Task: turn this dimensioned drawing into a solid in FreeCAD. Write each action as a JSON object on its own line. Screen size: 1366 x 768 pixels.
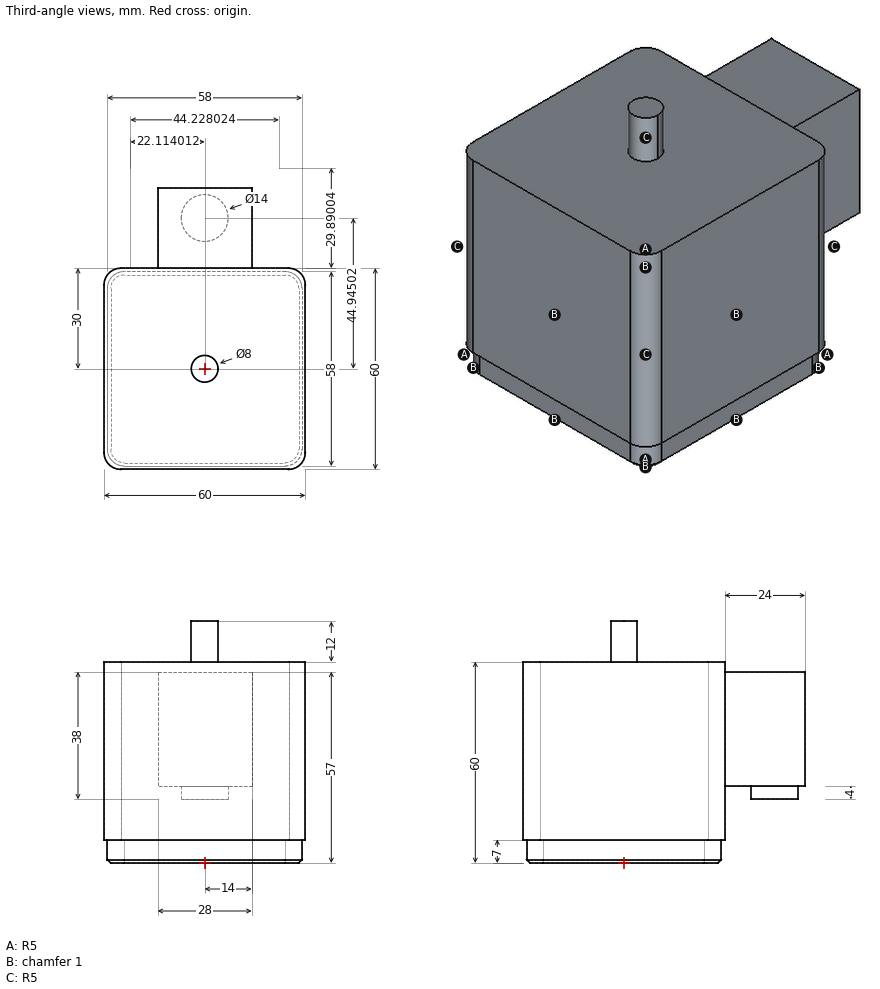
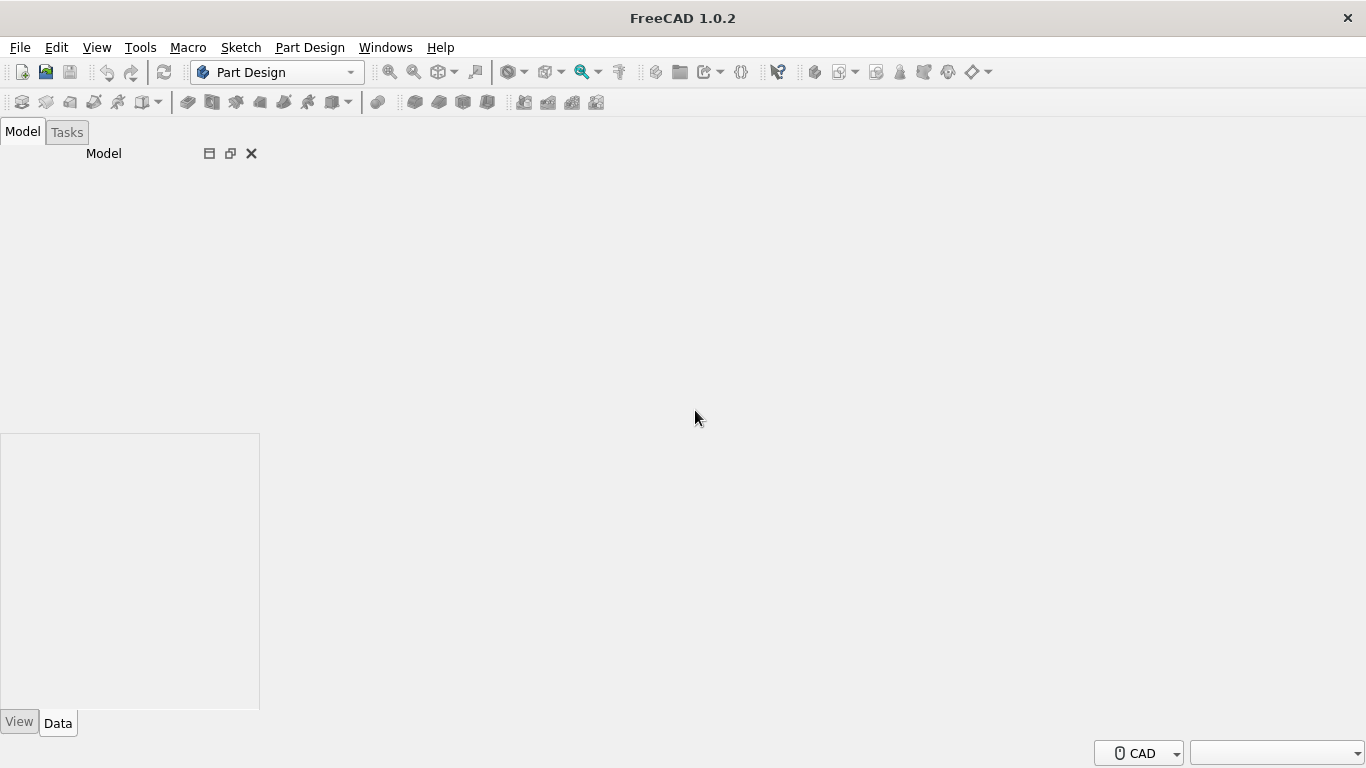
{"action": "key", "text": "ctrl+n"}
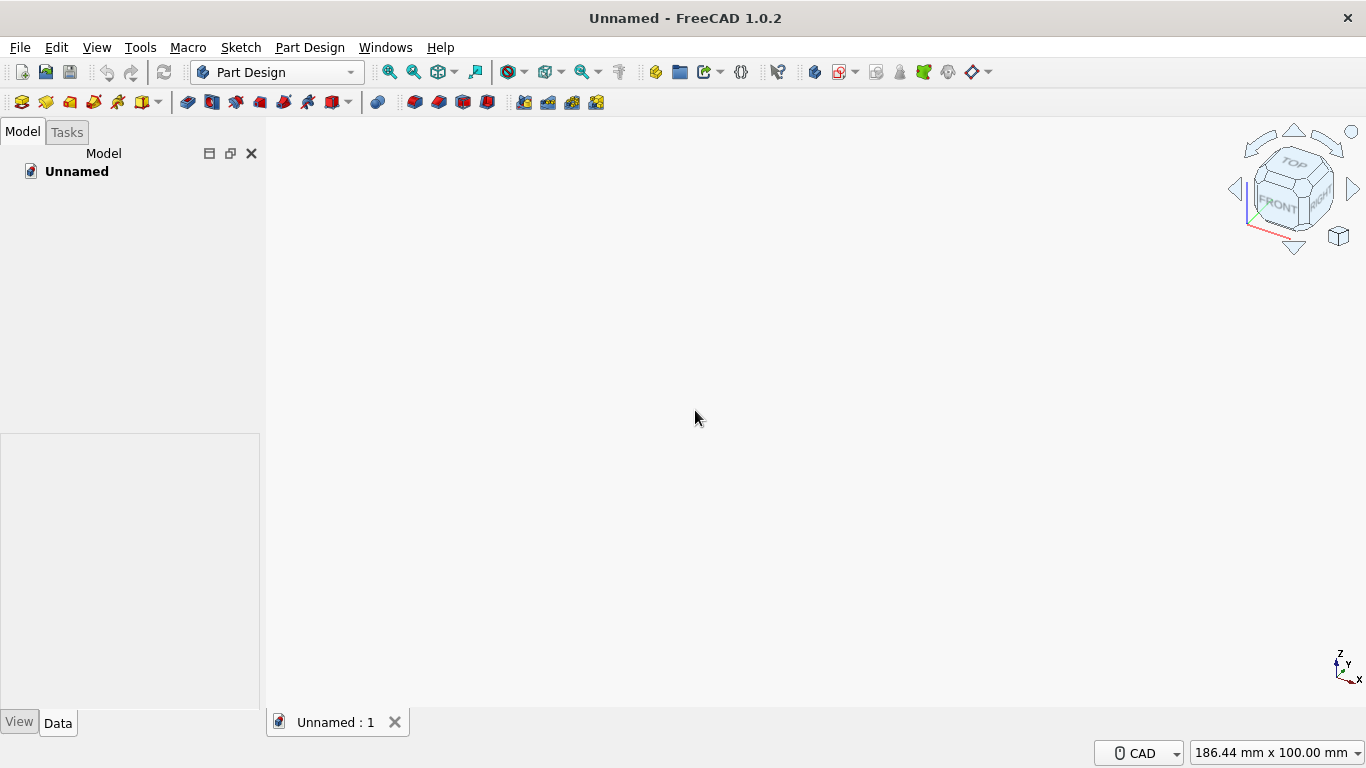
{"action": "left_click", "coordinate": [840, 72]}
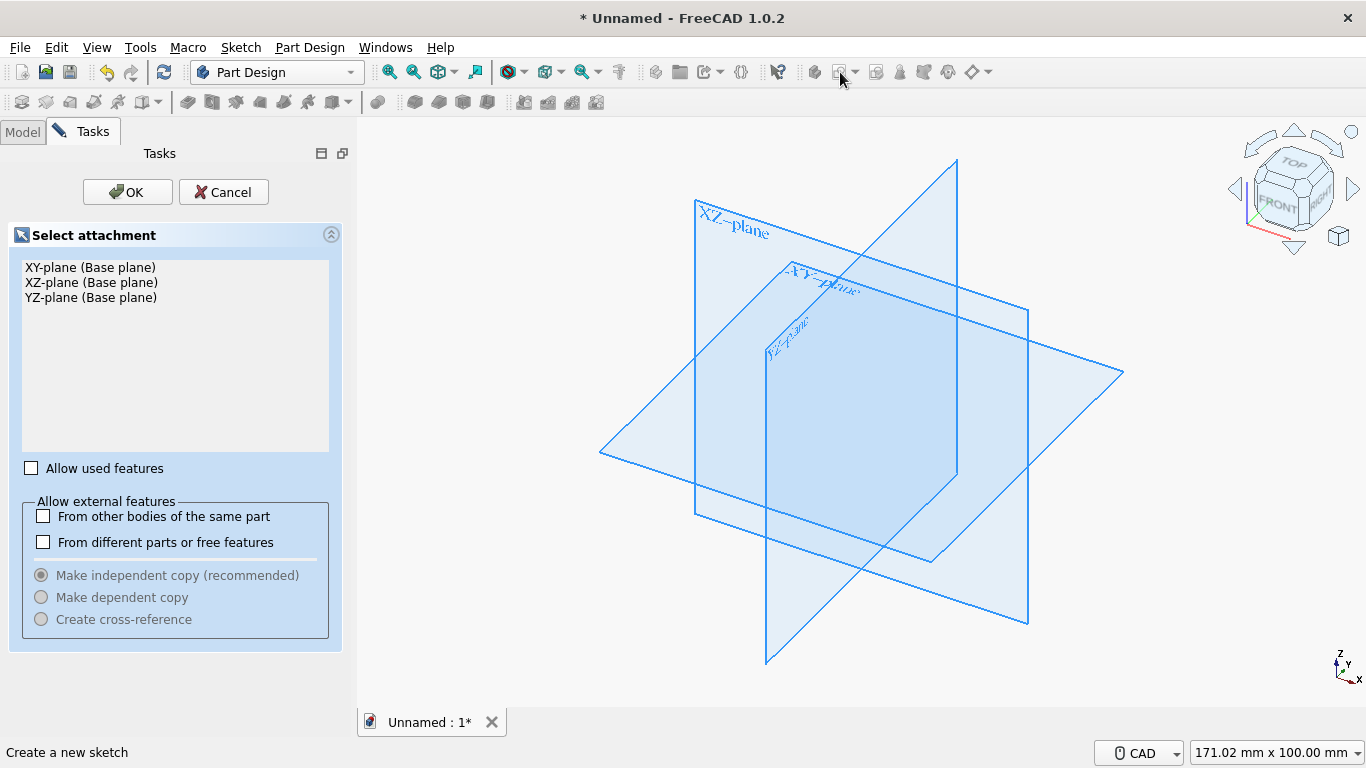
{"action": "left_click", "coordinate": [82, 268]}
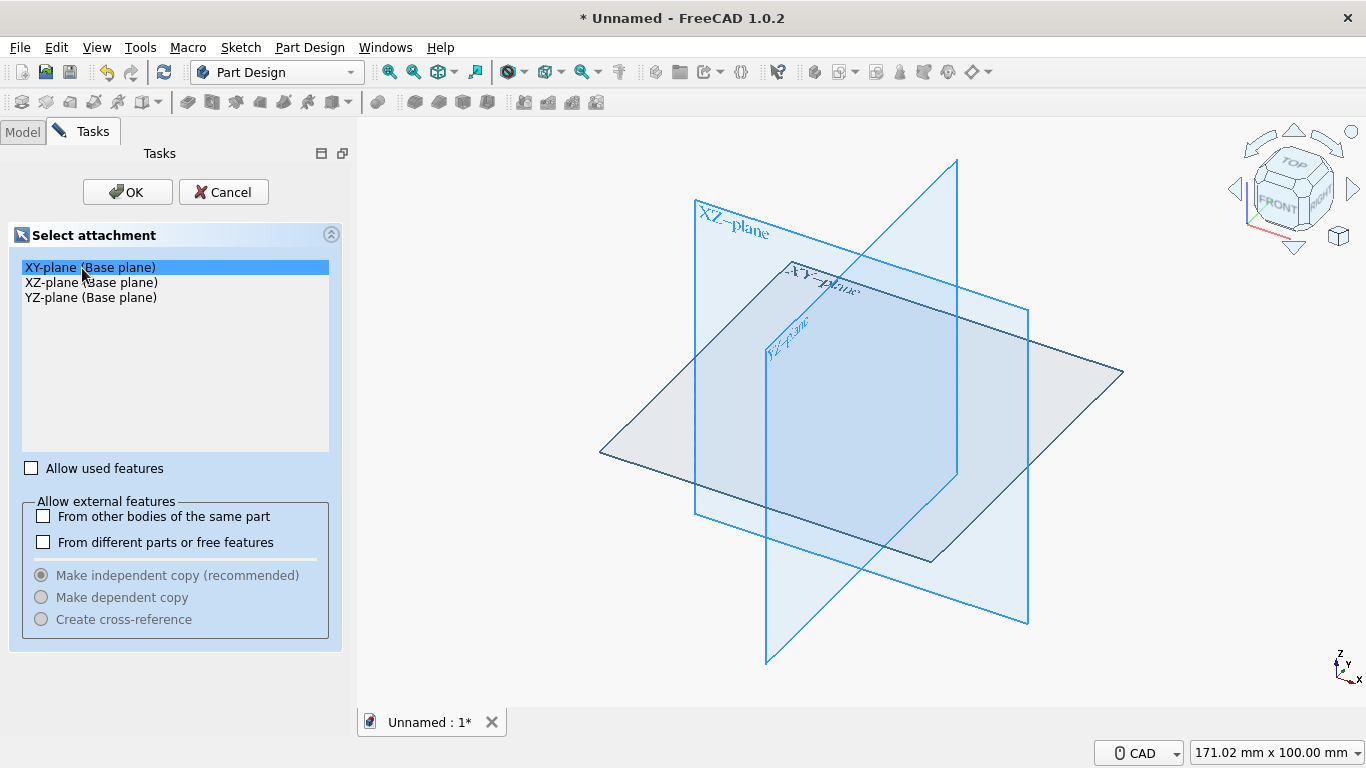
{"action": "left_click", "coordinate": [128, 192]}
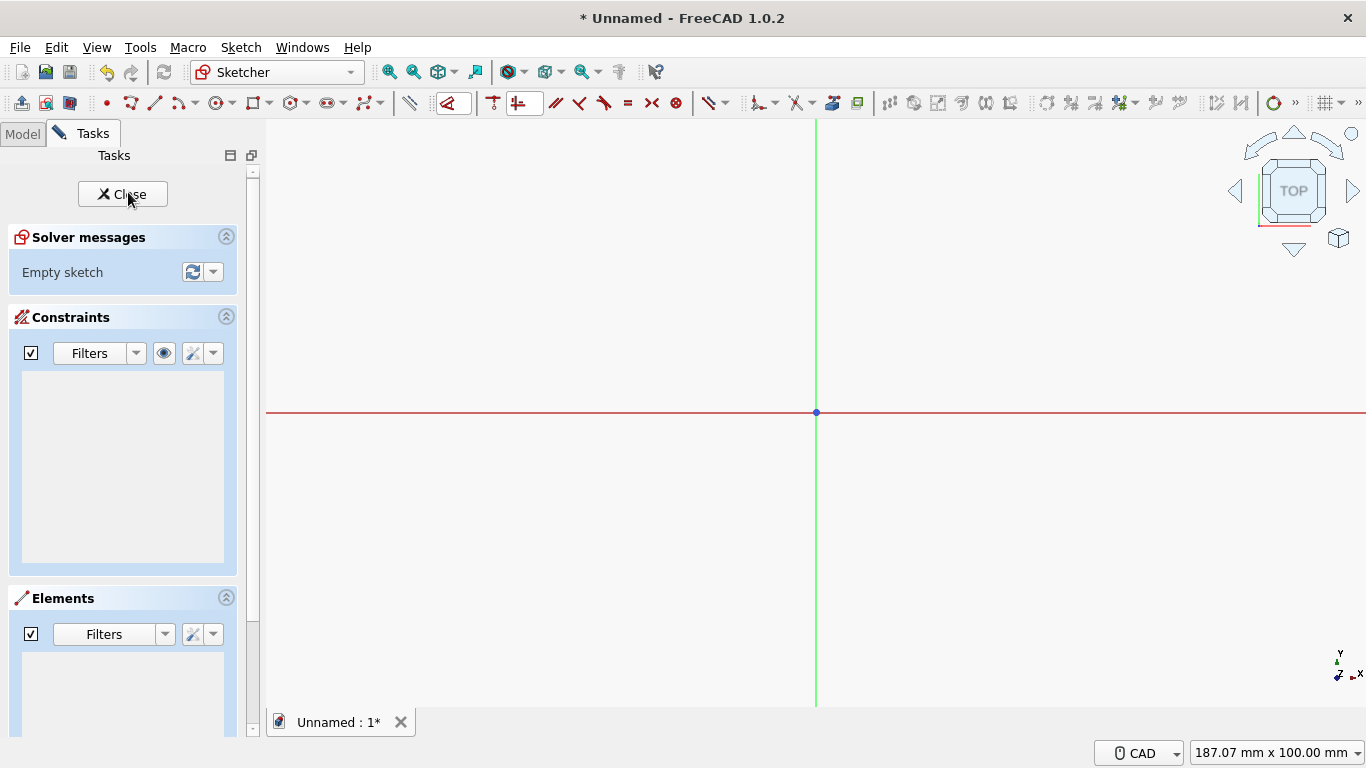
{"action": "key", "text": "g v"}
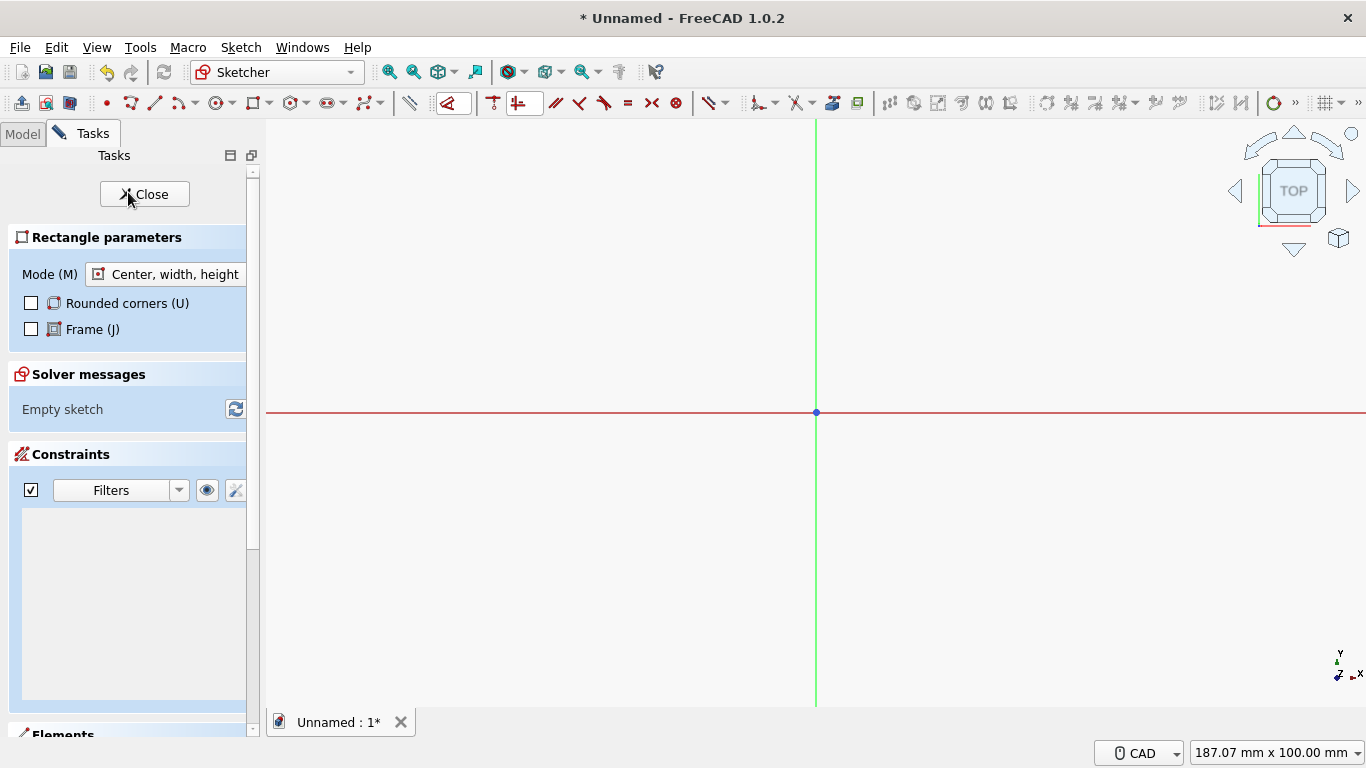
{"action": "left_click", "coordinate": [816, 413]}
{"action": "mouse_move", "coordinate": [992, 237]}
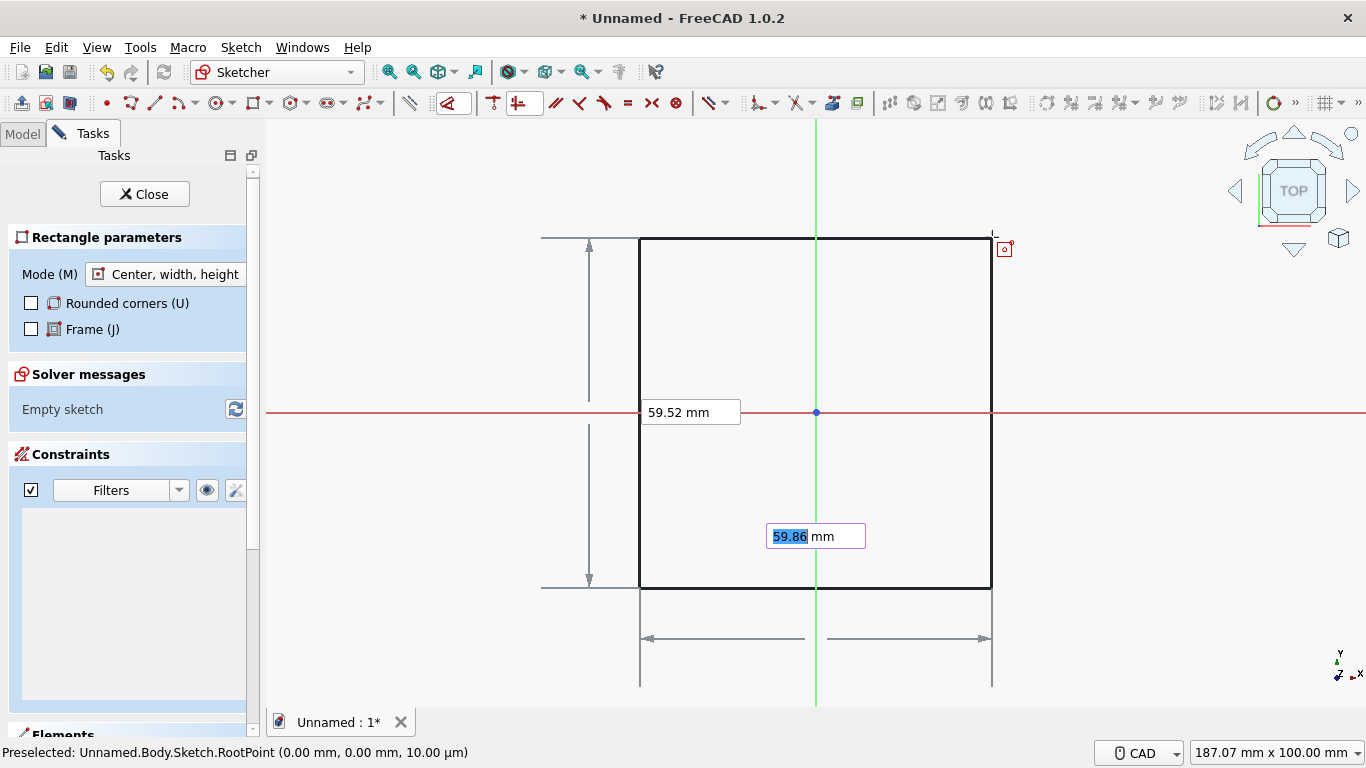
{"action": "type", "text": "60"}
{"action": "key", "text": "Tab"}
{"action": "type", "text": "60"}
{"action": "key", "text": "Return"}
{"action": "key", "text": "Escape"}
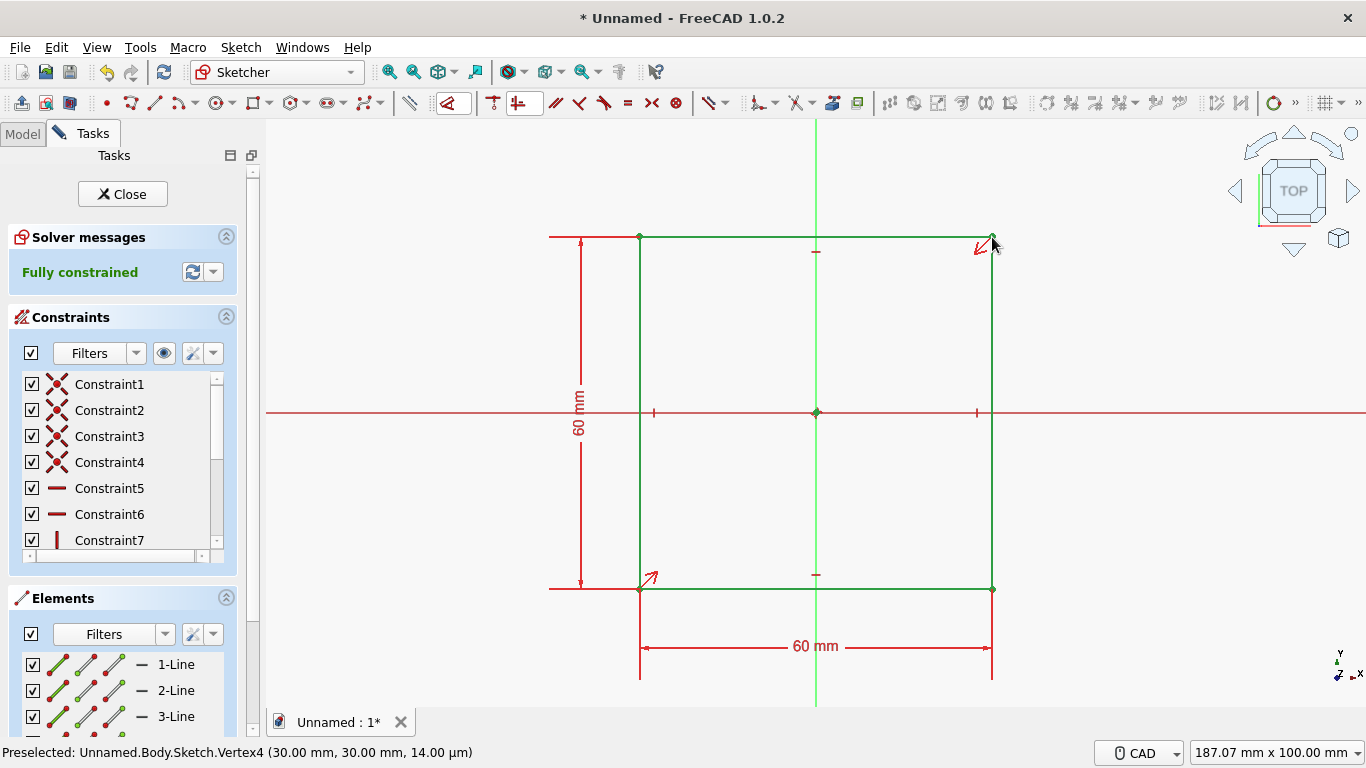
{"action": "left_click", "coordinate": [123, 194]}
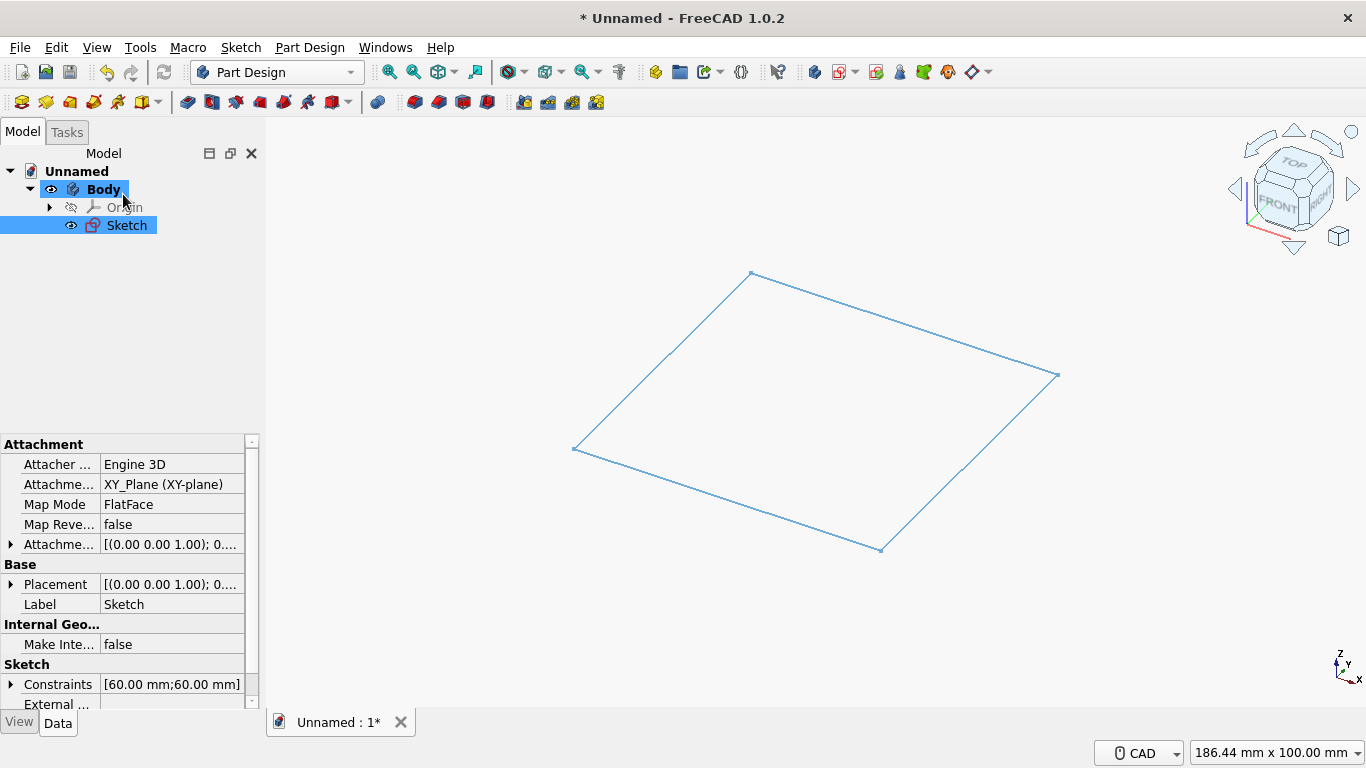
{"action": "left_click", "coordinate": [22, 102]}